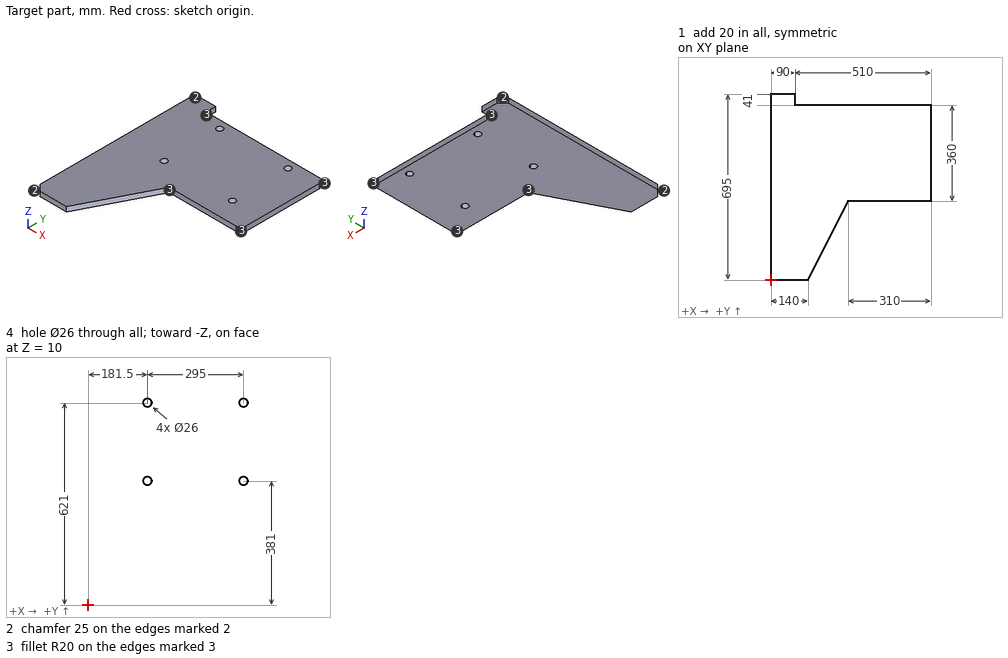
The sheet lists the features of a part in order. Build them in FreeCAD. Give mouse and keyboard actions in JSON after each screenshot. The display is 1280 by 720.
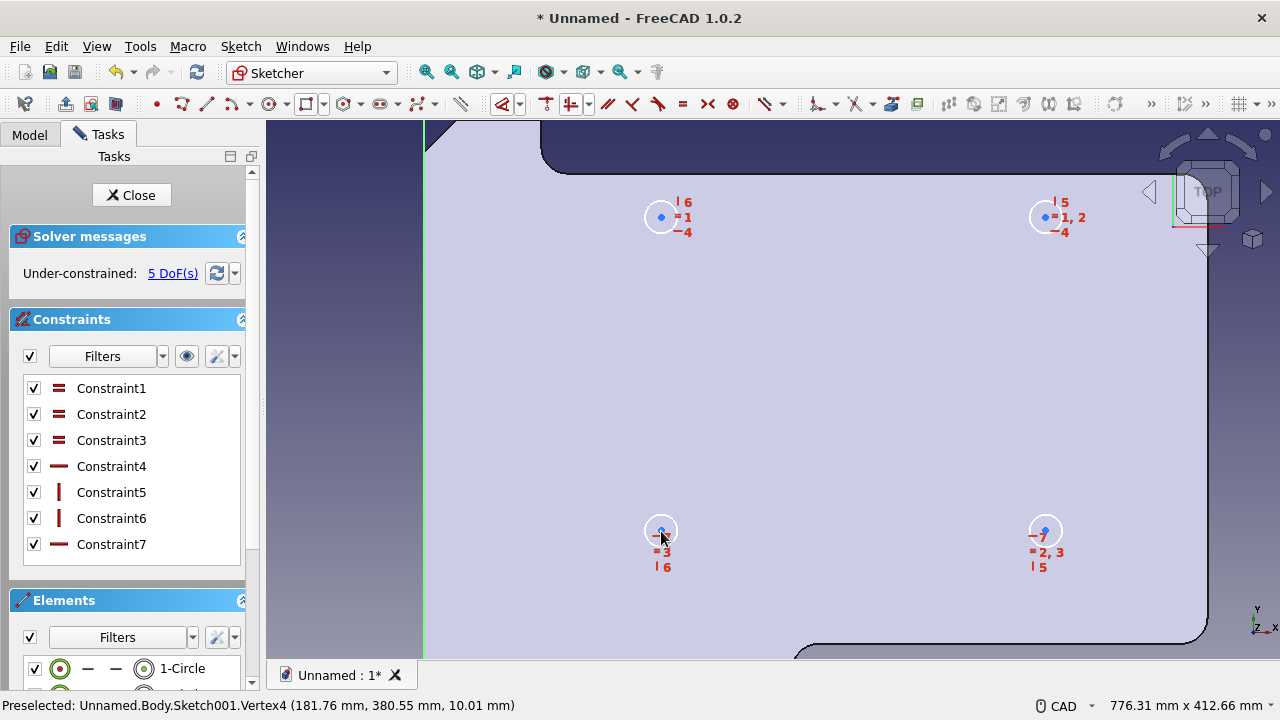
{"action": "left_click", "coordinate": [650, 206]}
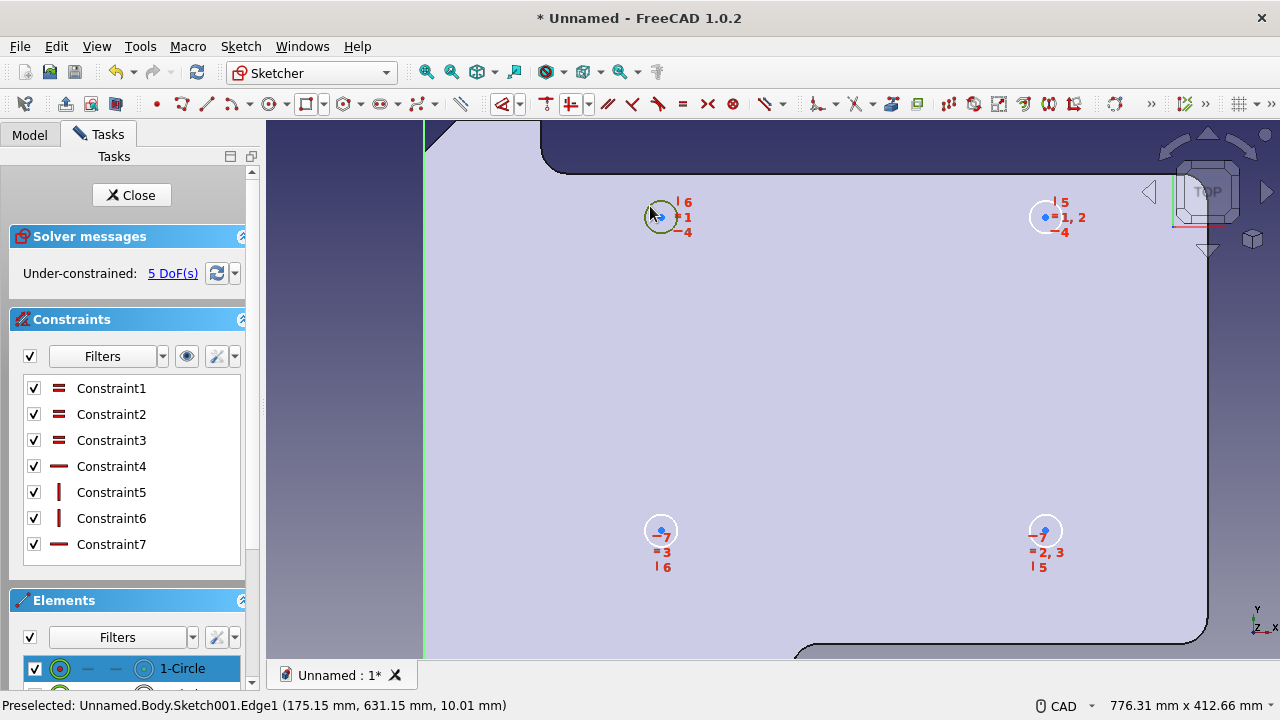
{"action": "left_click", "coordinate": [520, 104]}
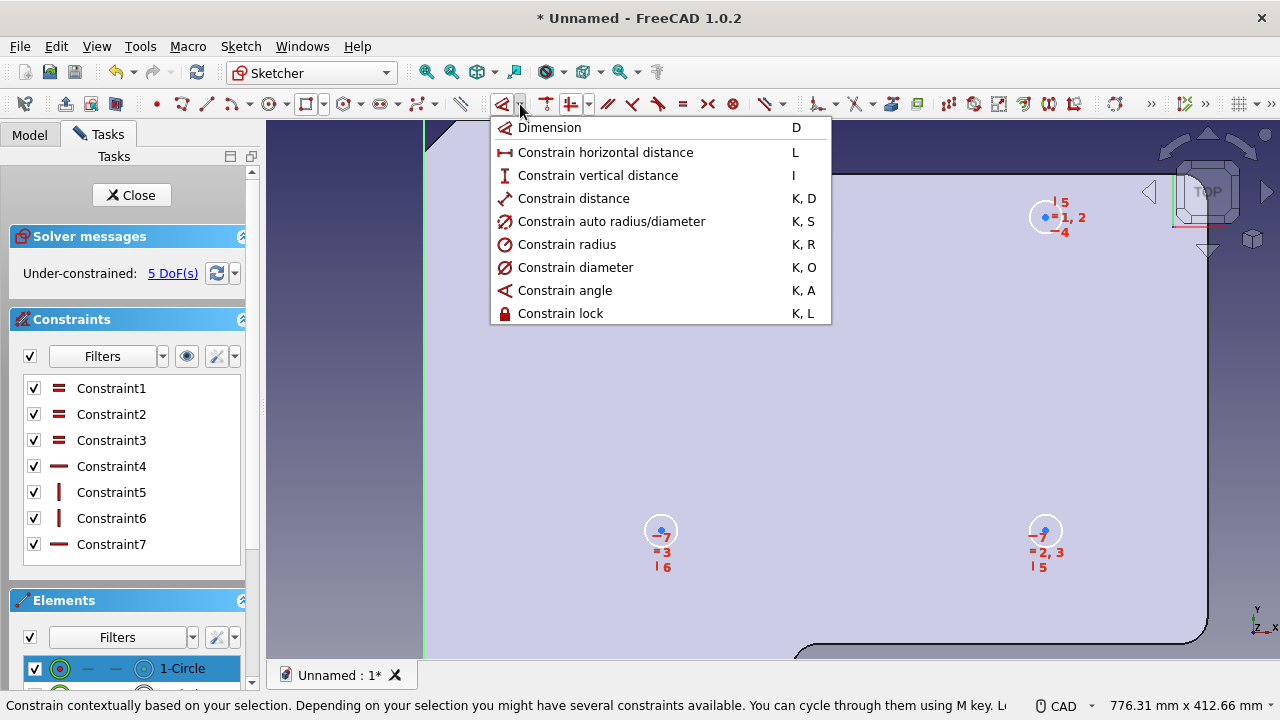
{"action": "left_click", "coordinate": [661, 268]}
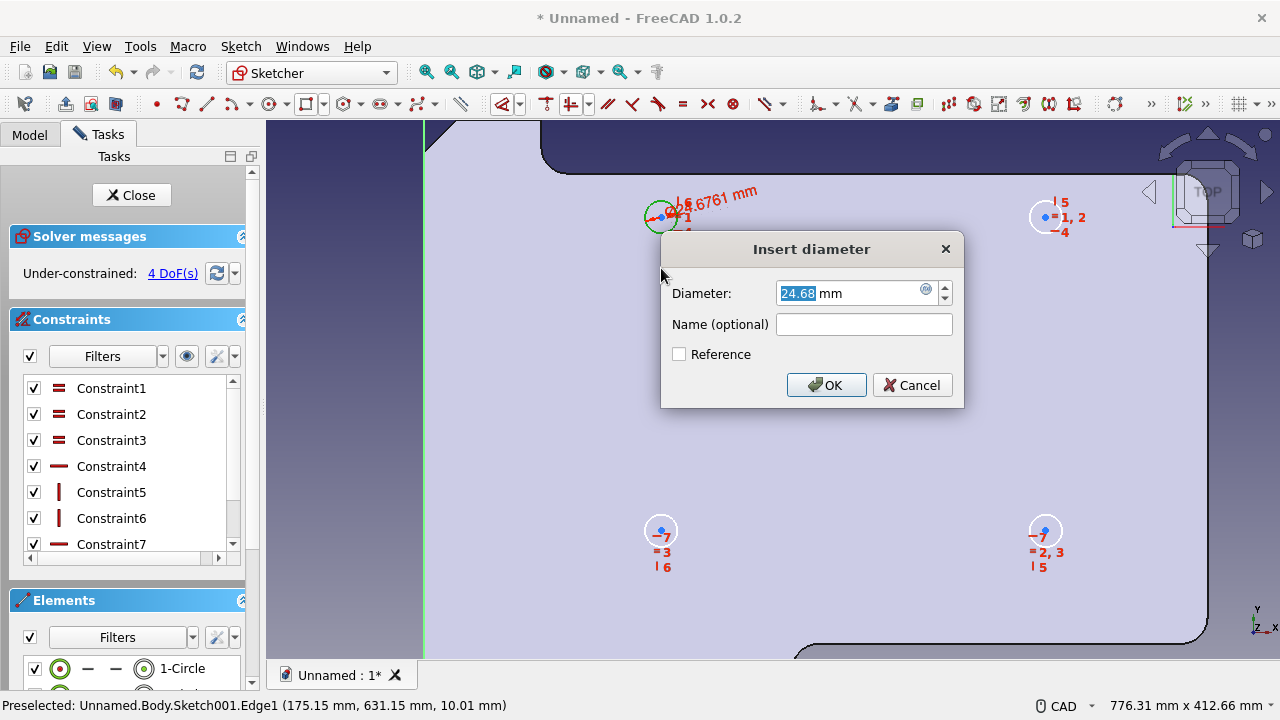
{"action": "type", "text": "26"}
{"action": "key", "text": "Return"}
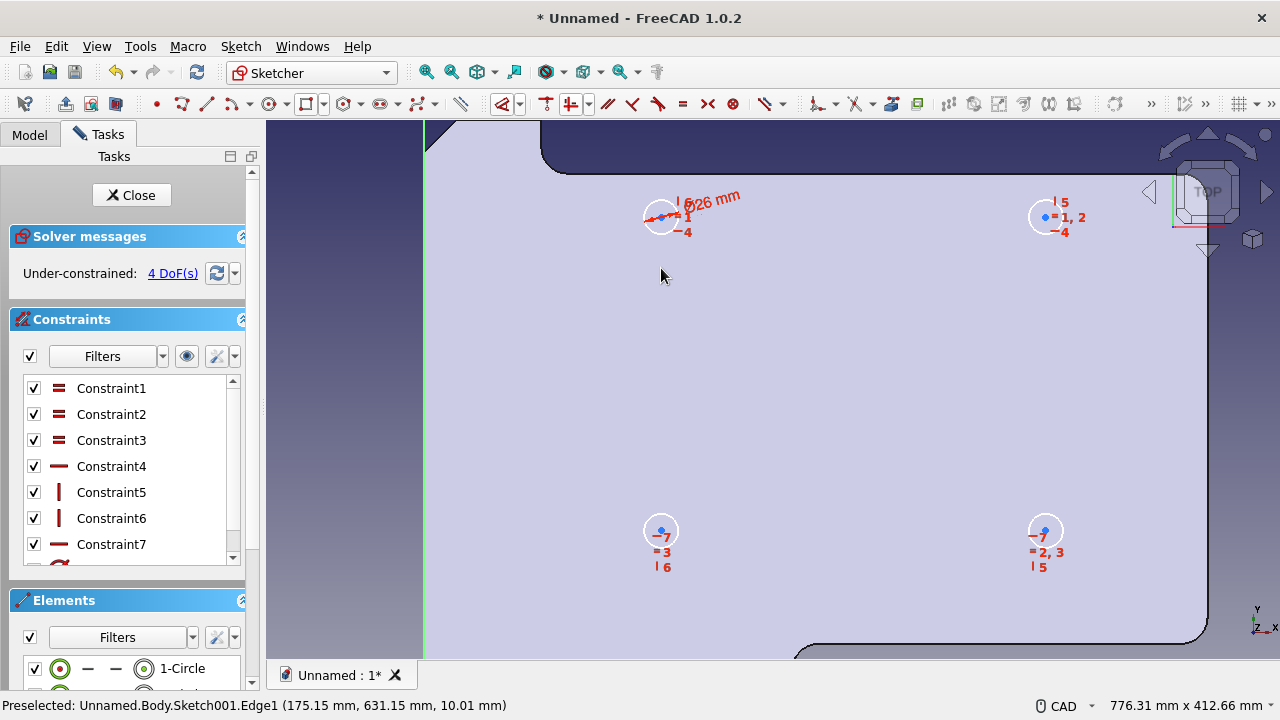
{"action": "left_click", "coordinate": [661, 217]}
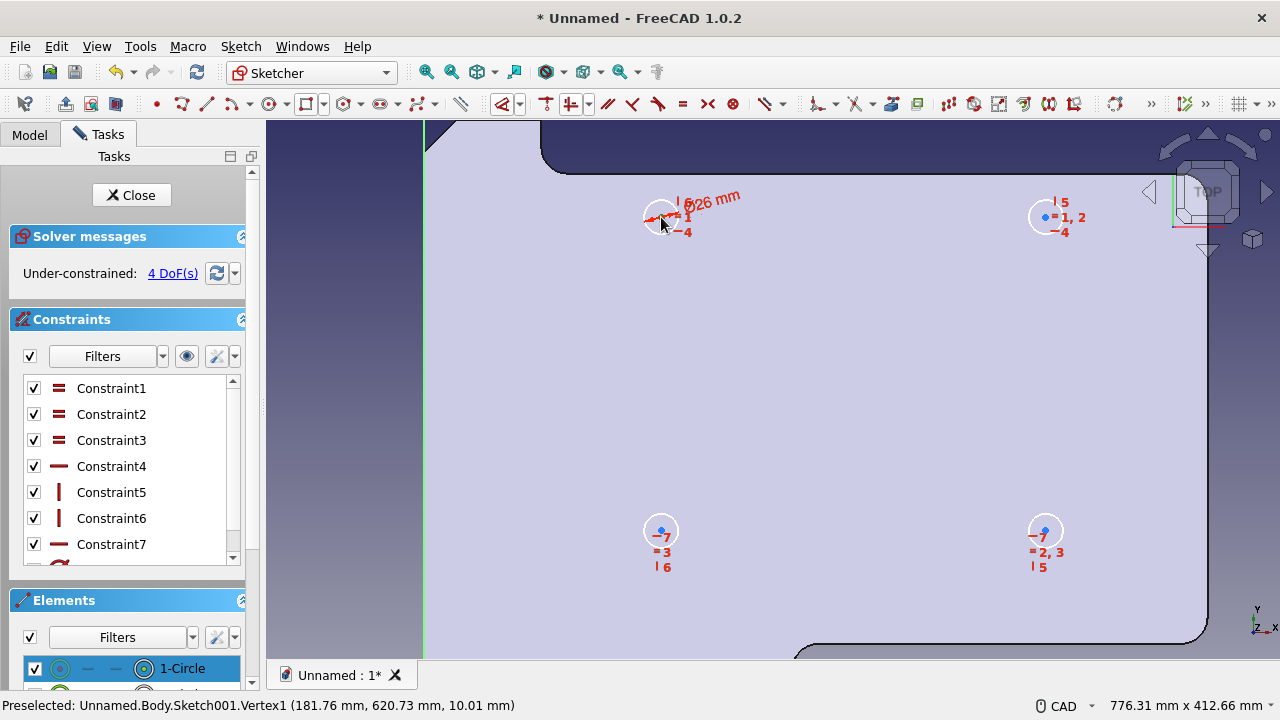
{"action": "left_click", "coordinate": [520, 104]}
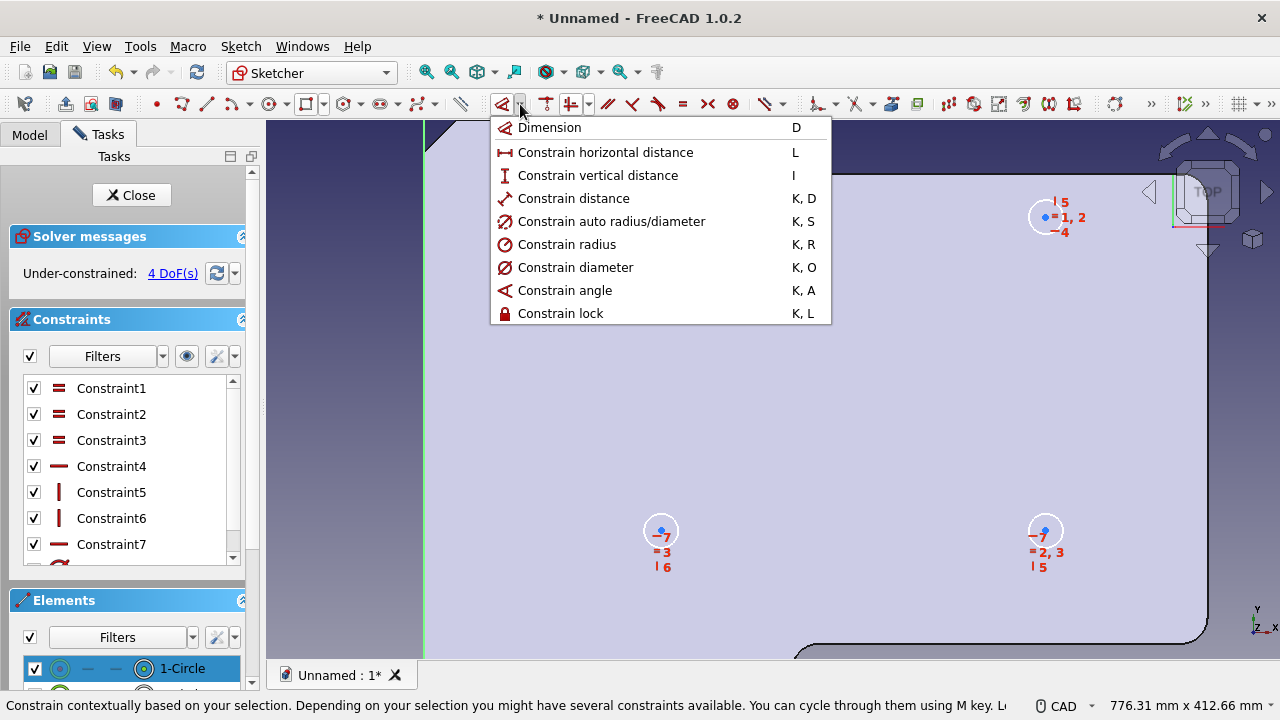
{"action": "left_click", "coordinate": [661, 176]}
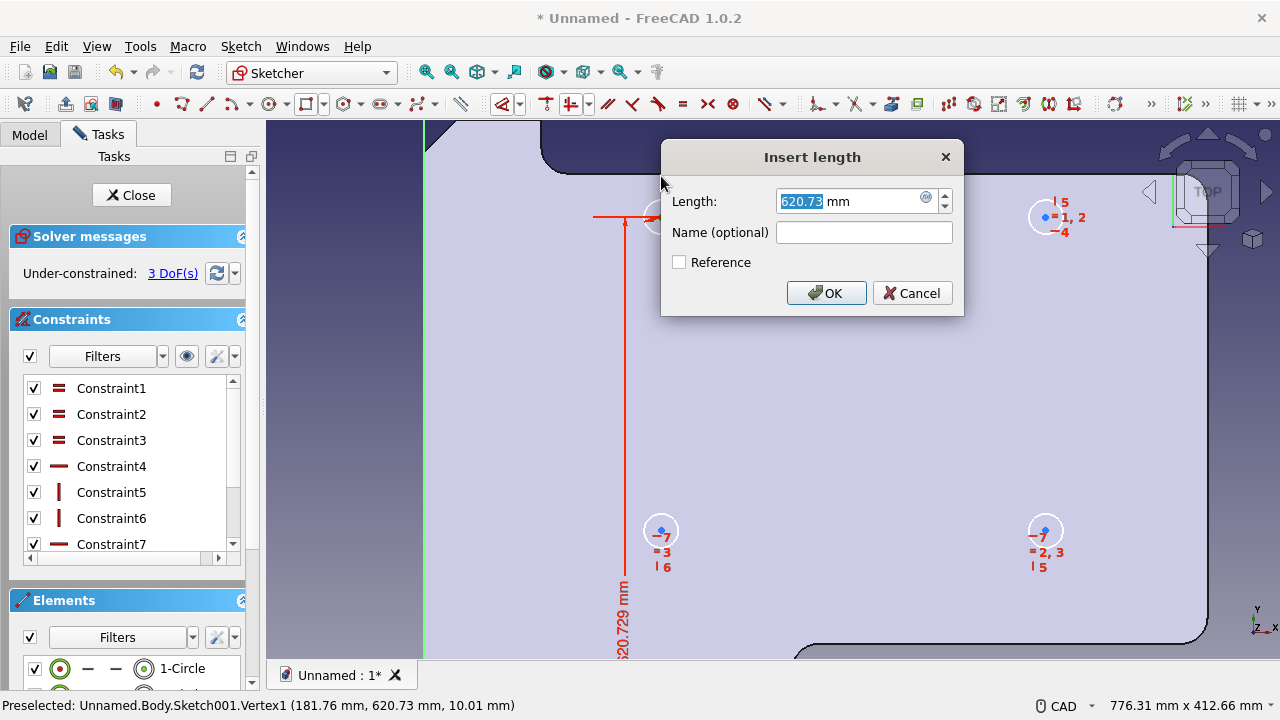
{"action": "type", "text": "621"}
{"action": "key", "text": "Return"}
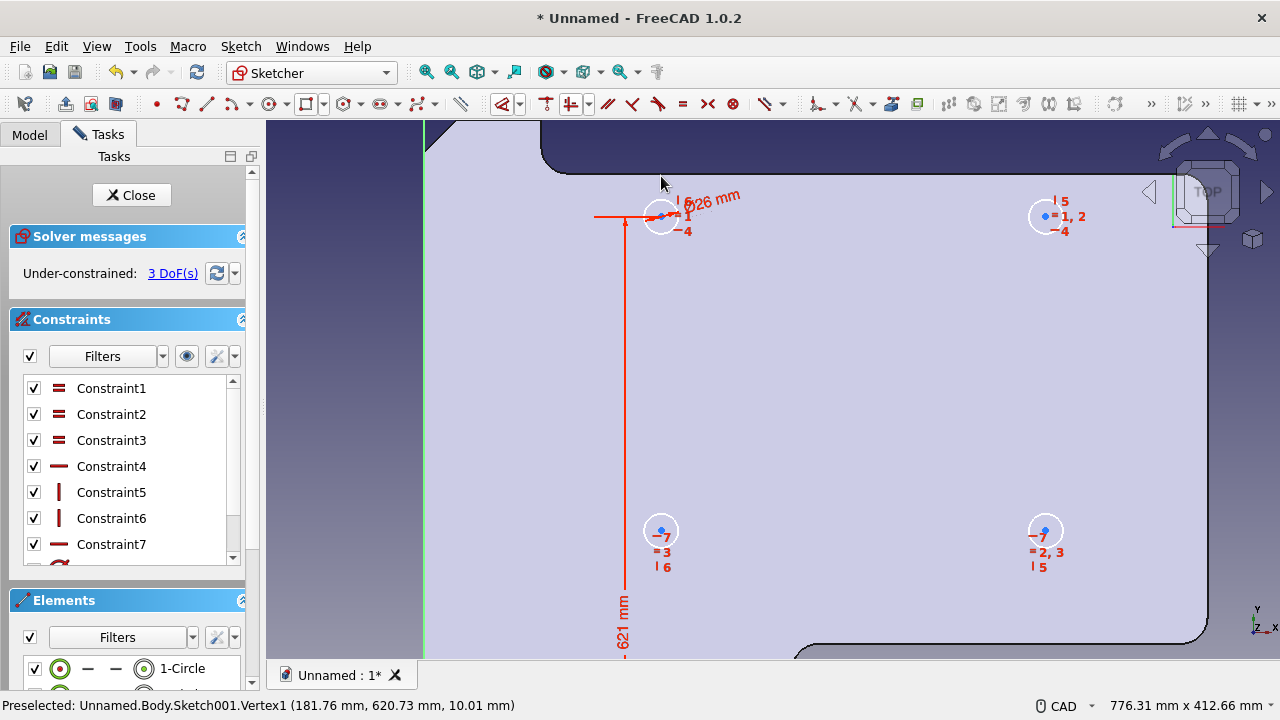
{"action": "left_click", "coordinate": [1046, 531]}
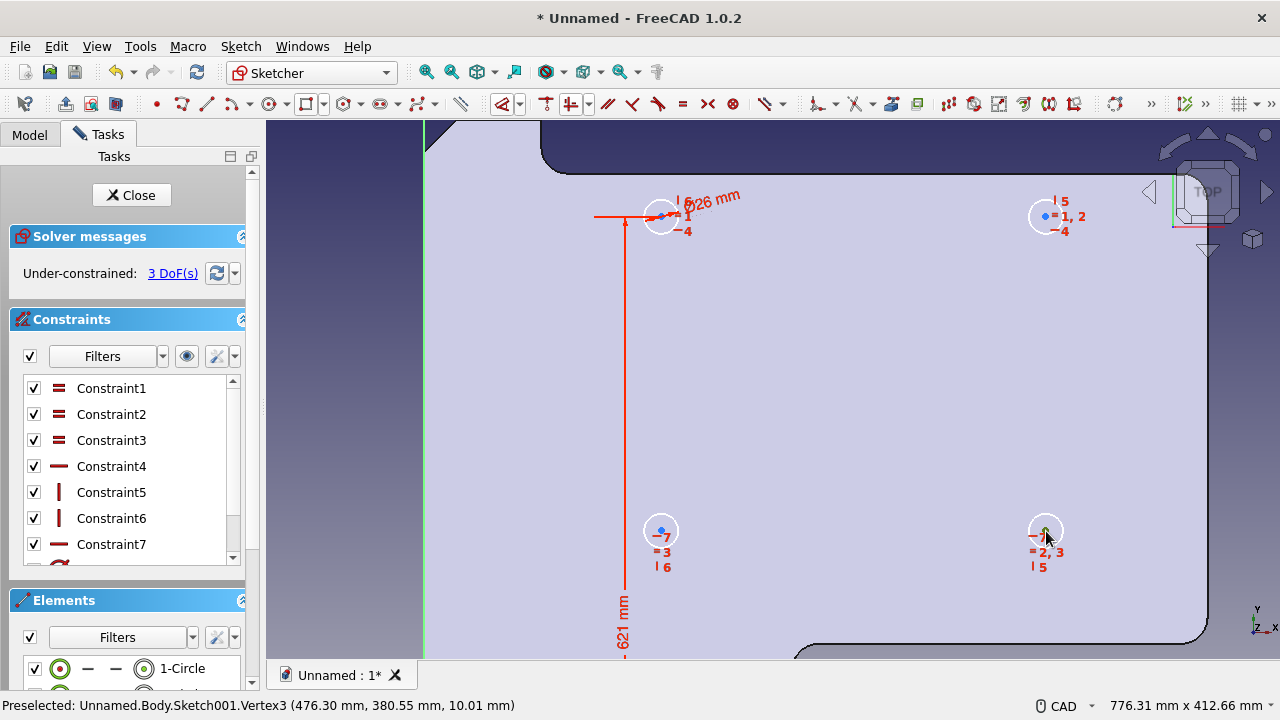
{"action": "left_click", "coordinate": [520, 104]}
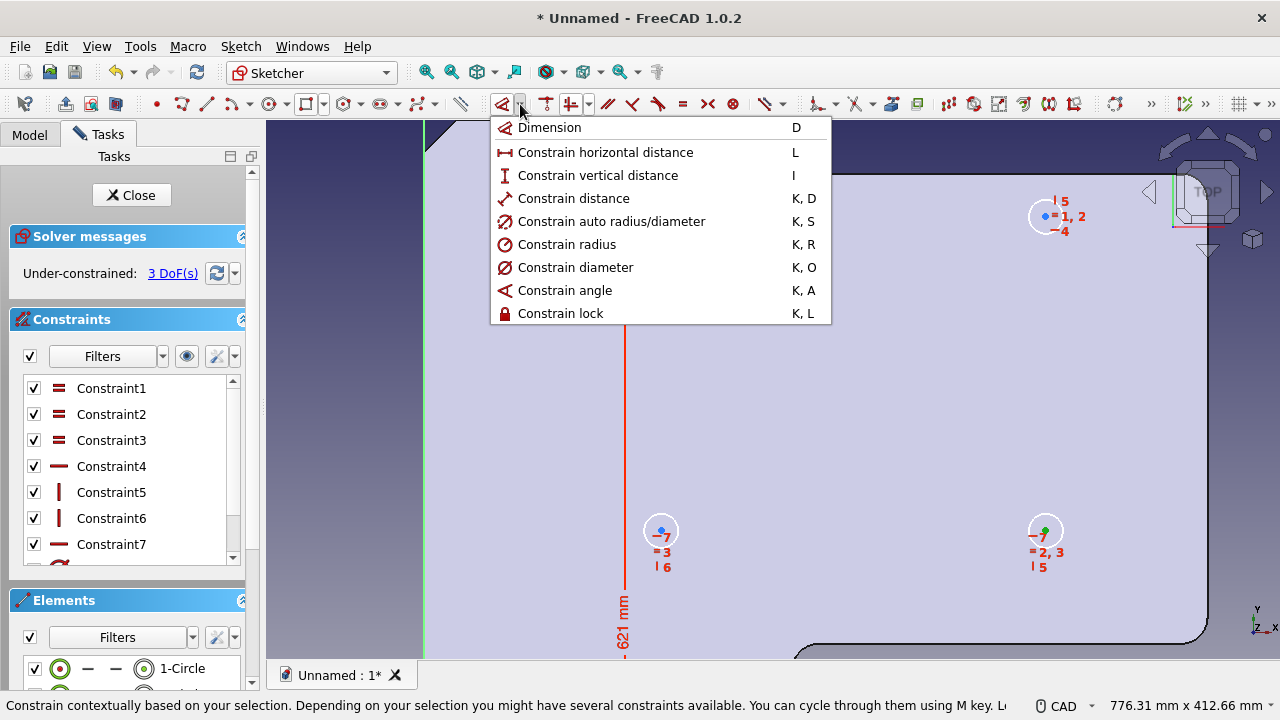
{"action": "left_click", "coordinate": [661, 176]}